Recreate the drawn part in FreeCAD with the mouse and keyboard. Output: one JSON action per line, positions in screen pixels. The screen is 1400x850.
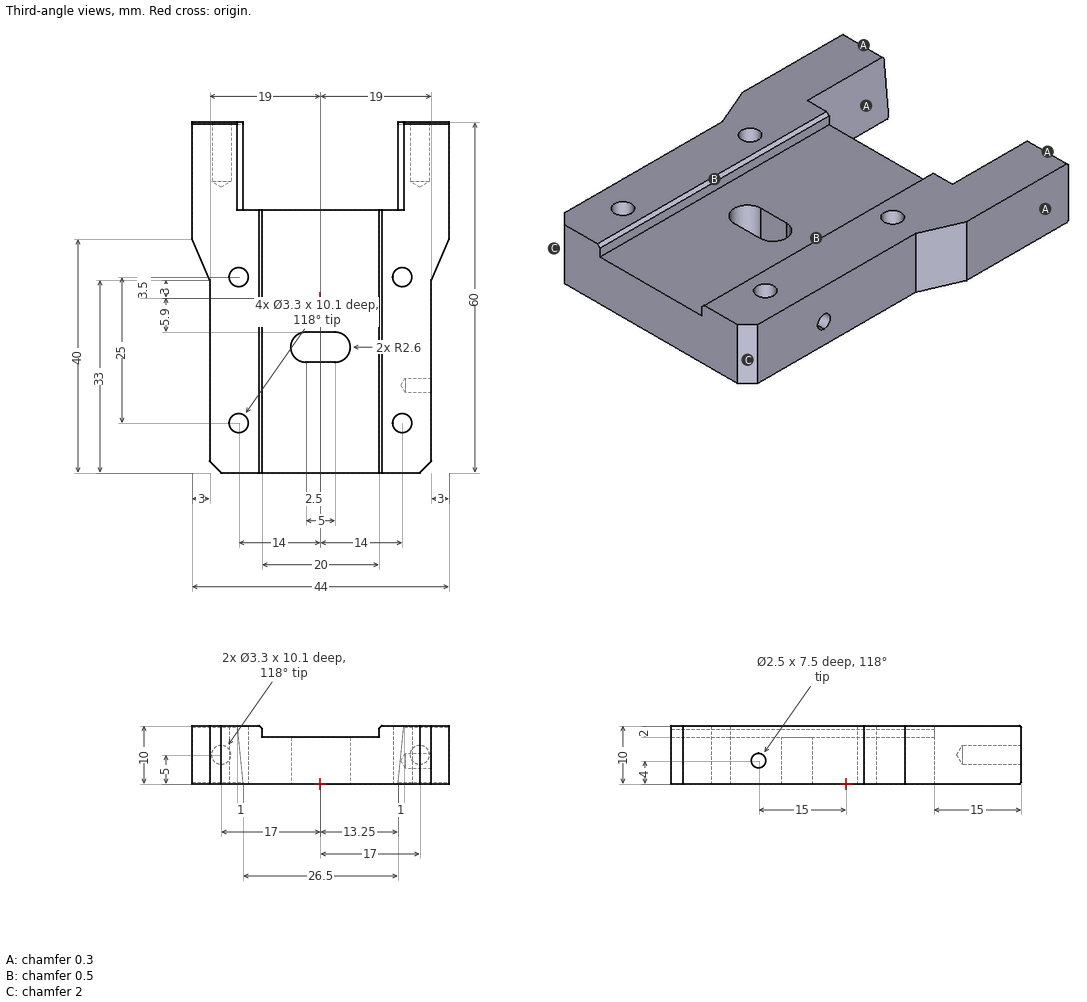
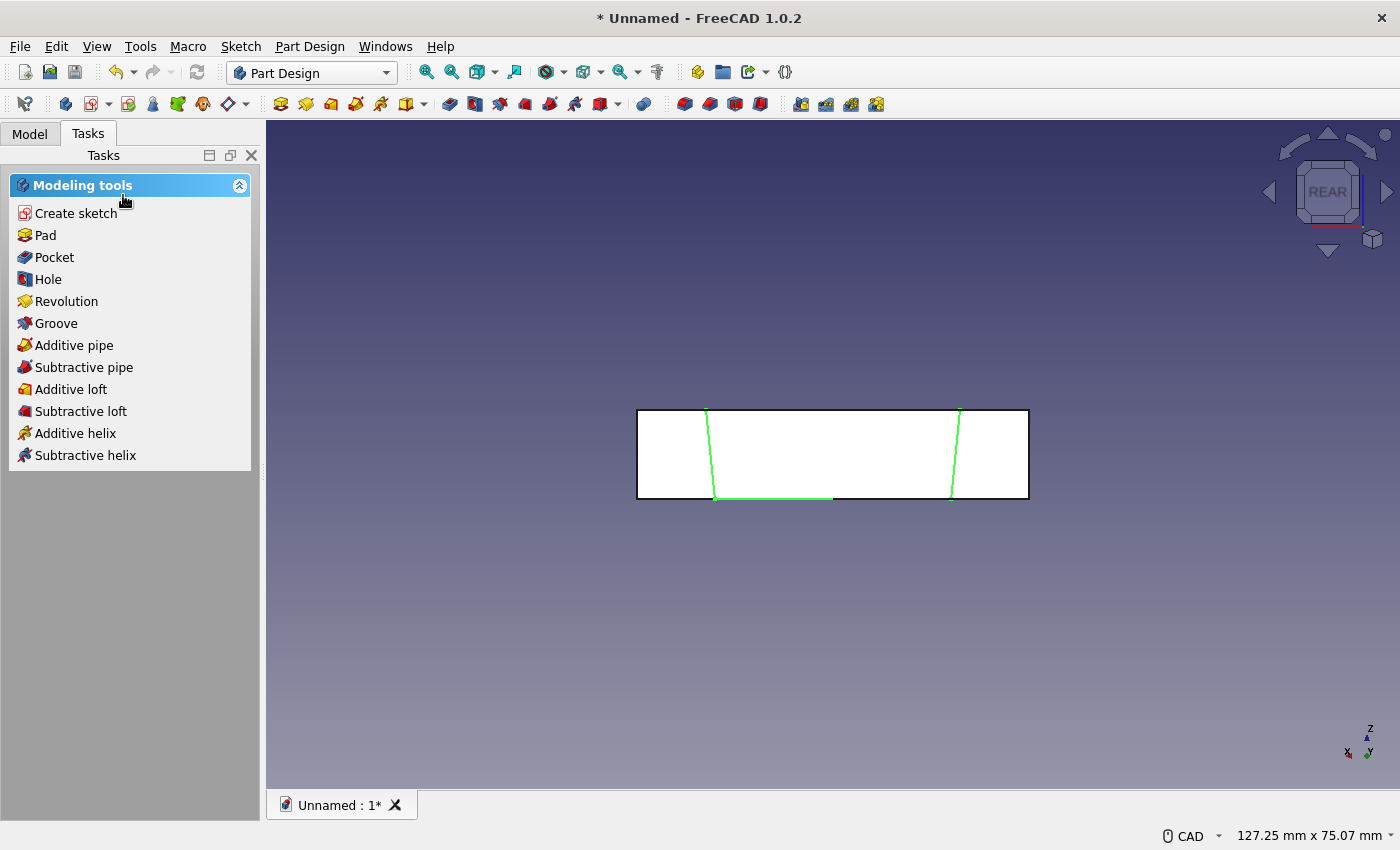
{"action": "left_click", "coordinate": [450, 104]}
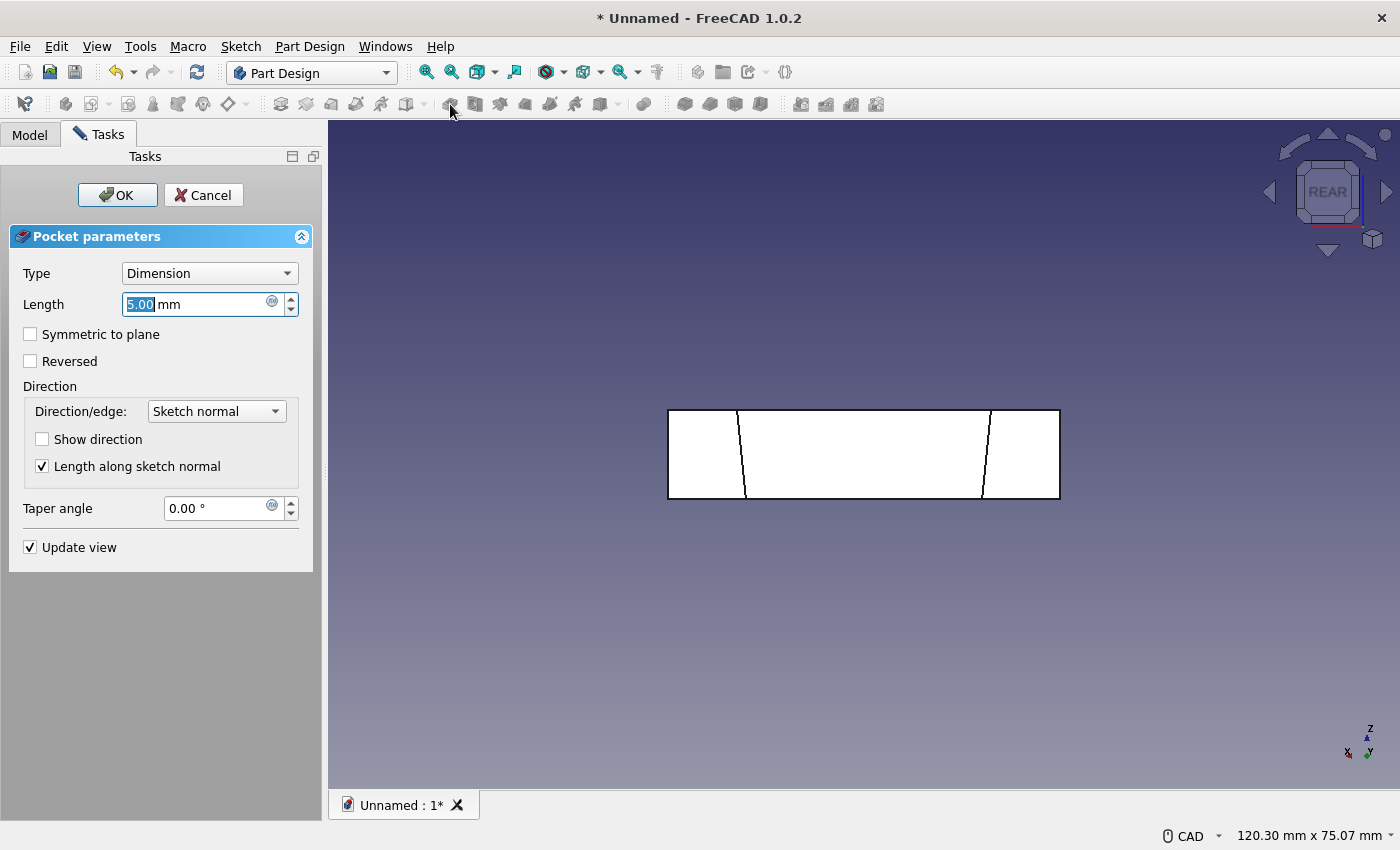
{"action": "type", "text": "15"}
{"action": "key", "text": "Tab"}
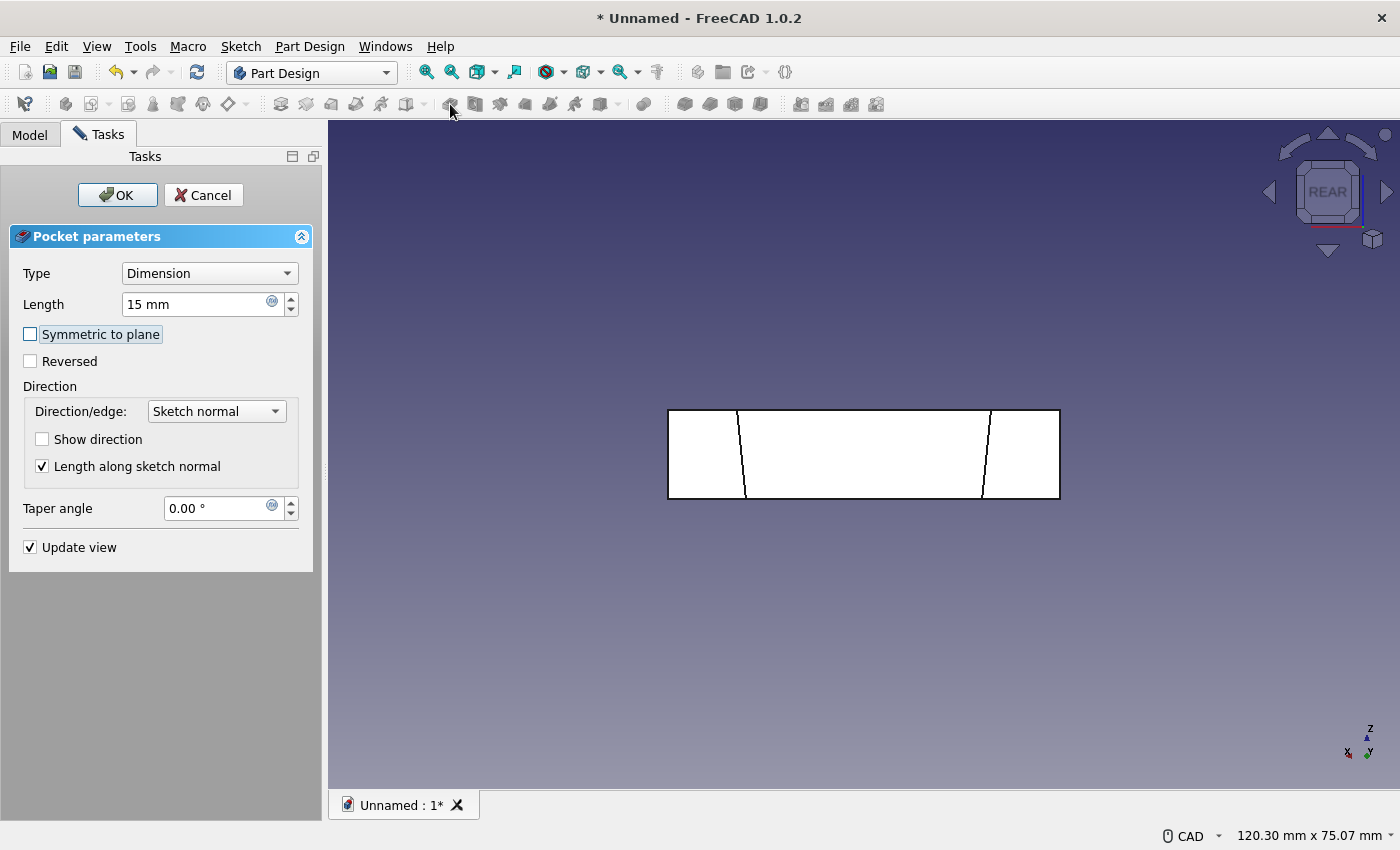
{"action": "left_click", "coordinate": [118, 195]}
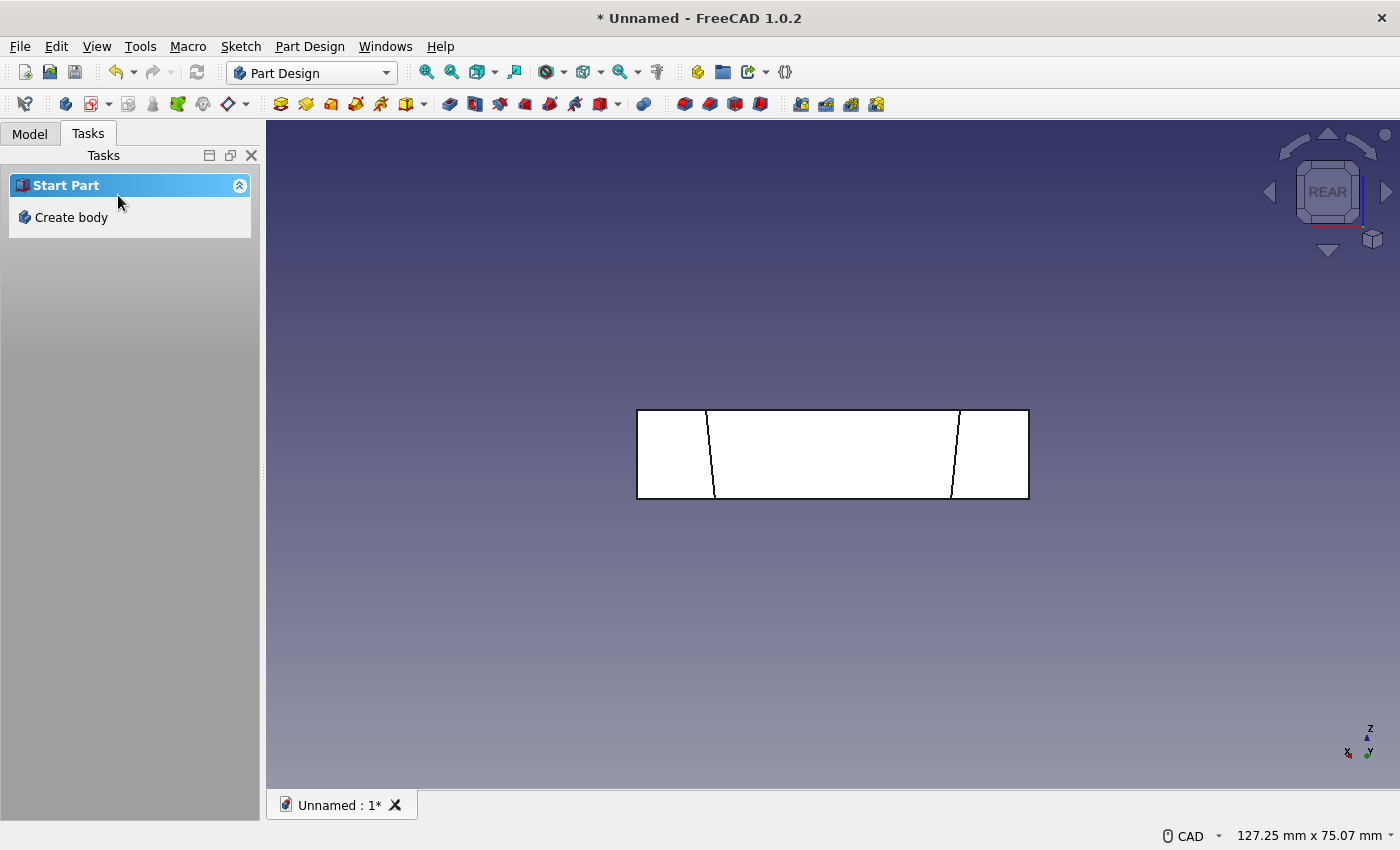
{"action": "left_click", "coordinate": [427, 72]}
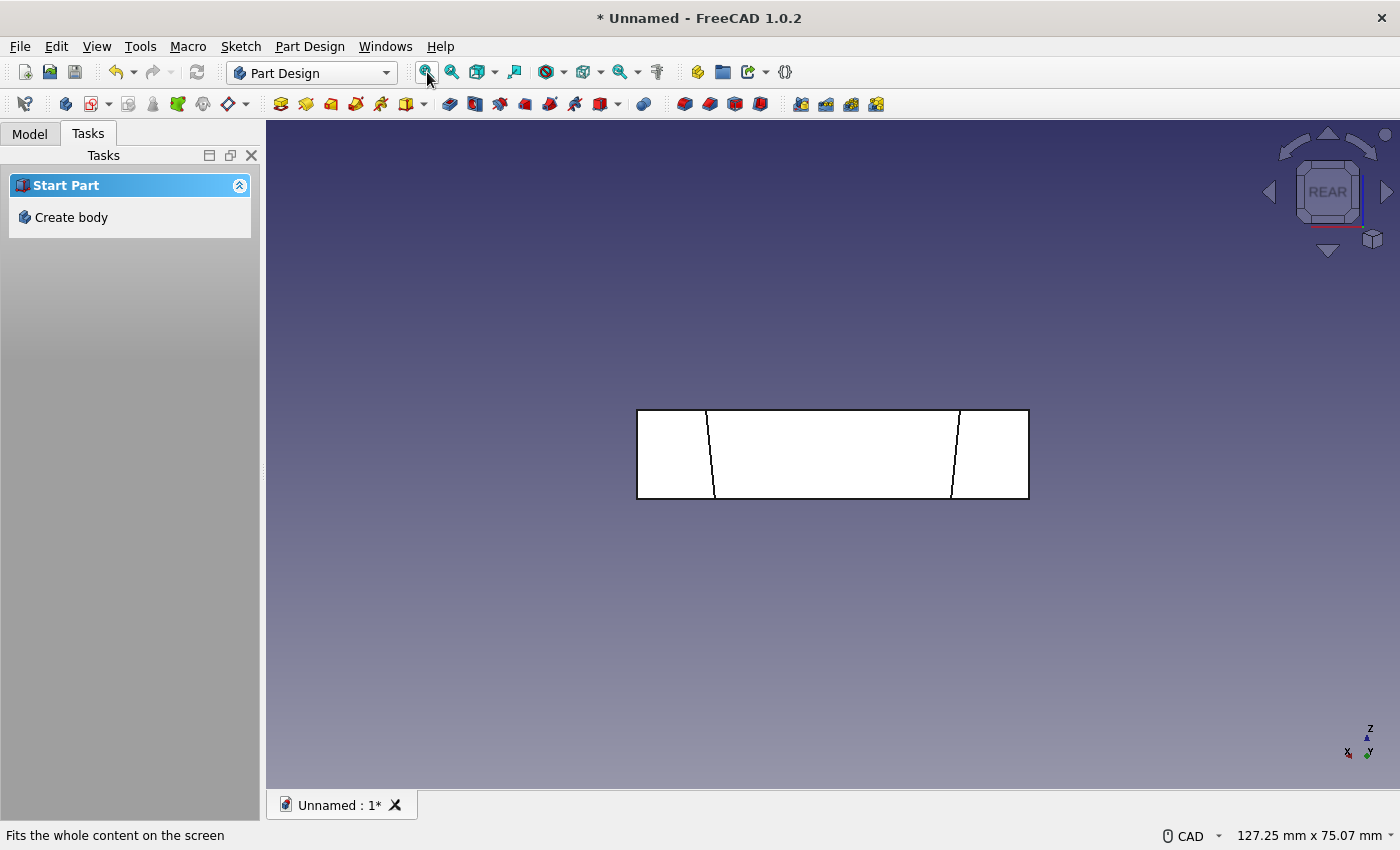
{"action": "key", "text": "0"}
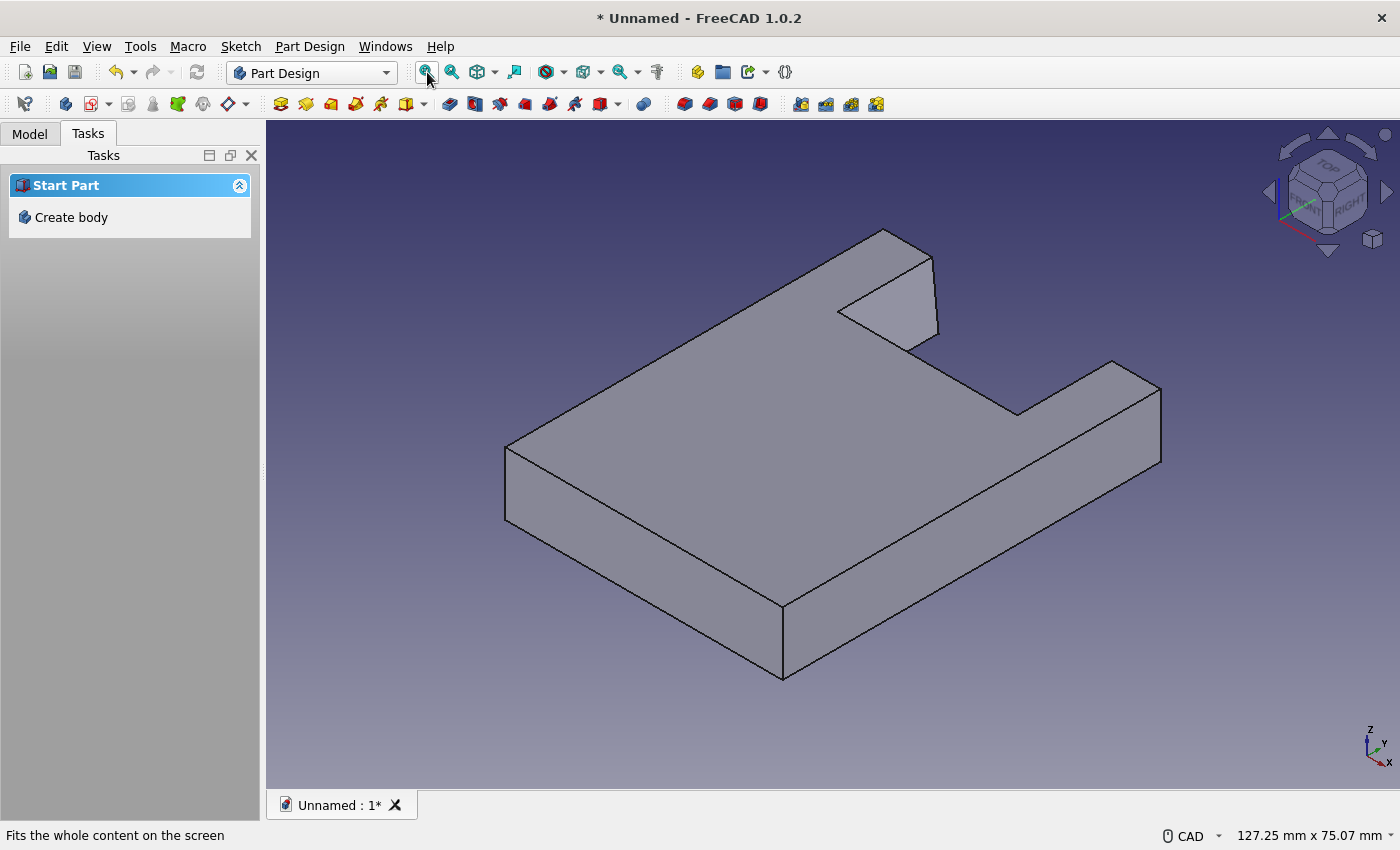
{"action": "left_click", "coordinate": [779, 448]}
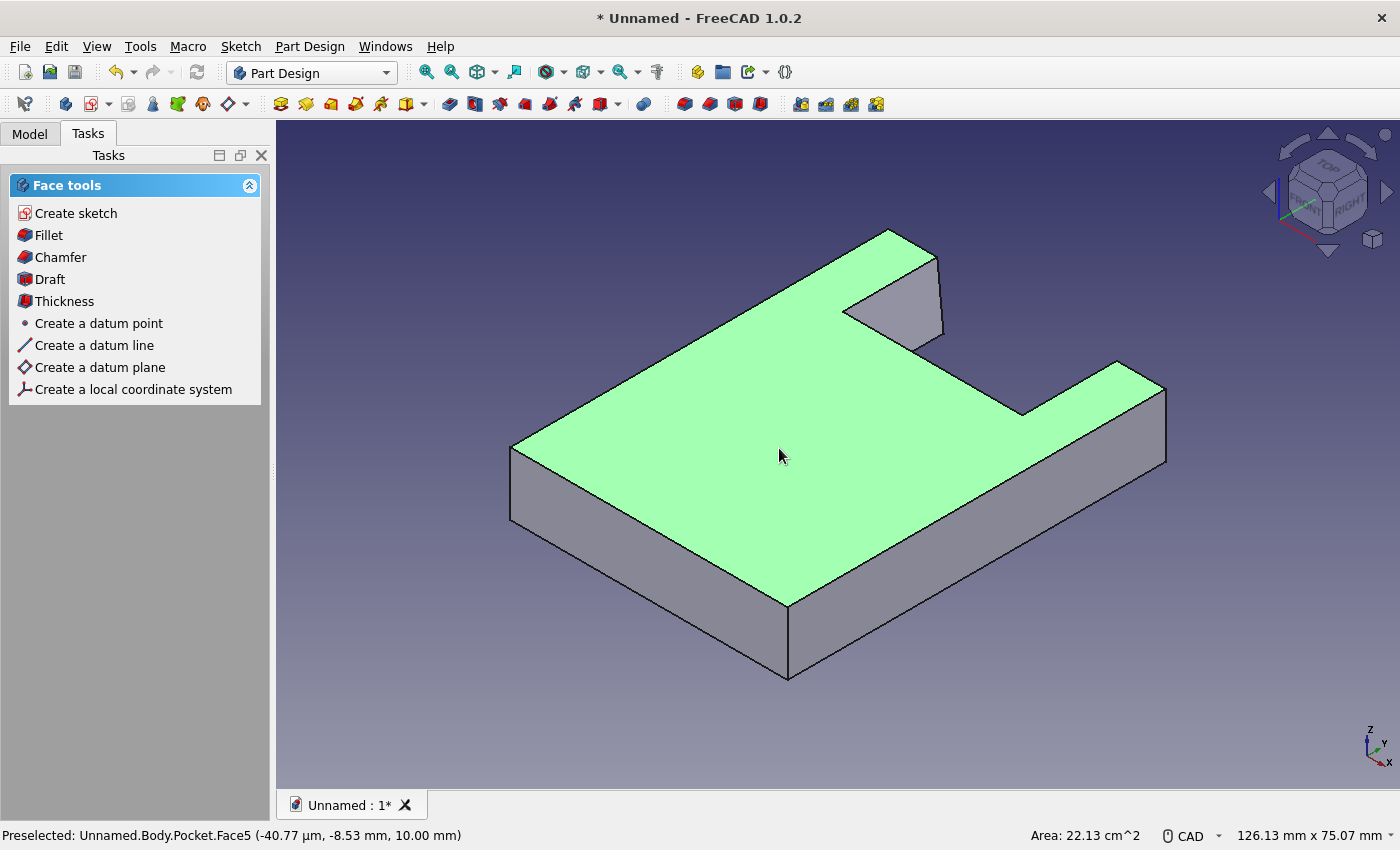
{"action": "left_click", "coordinate": [90, 104]}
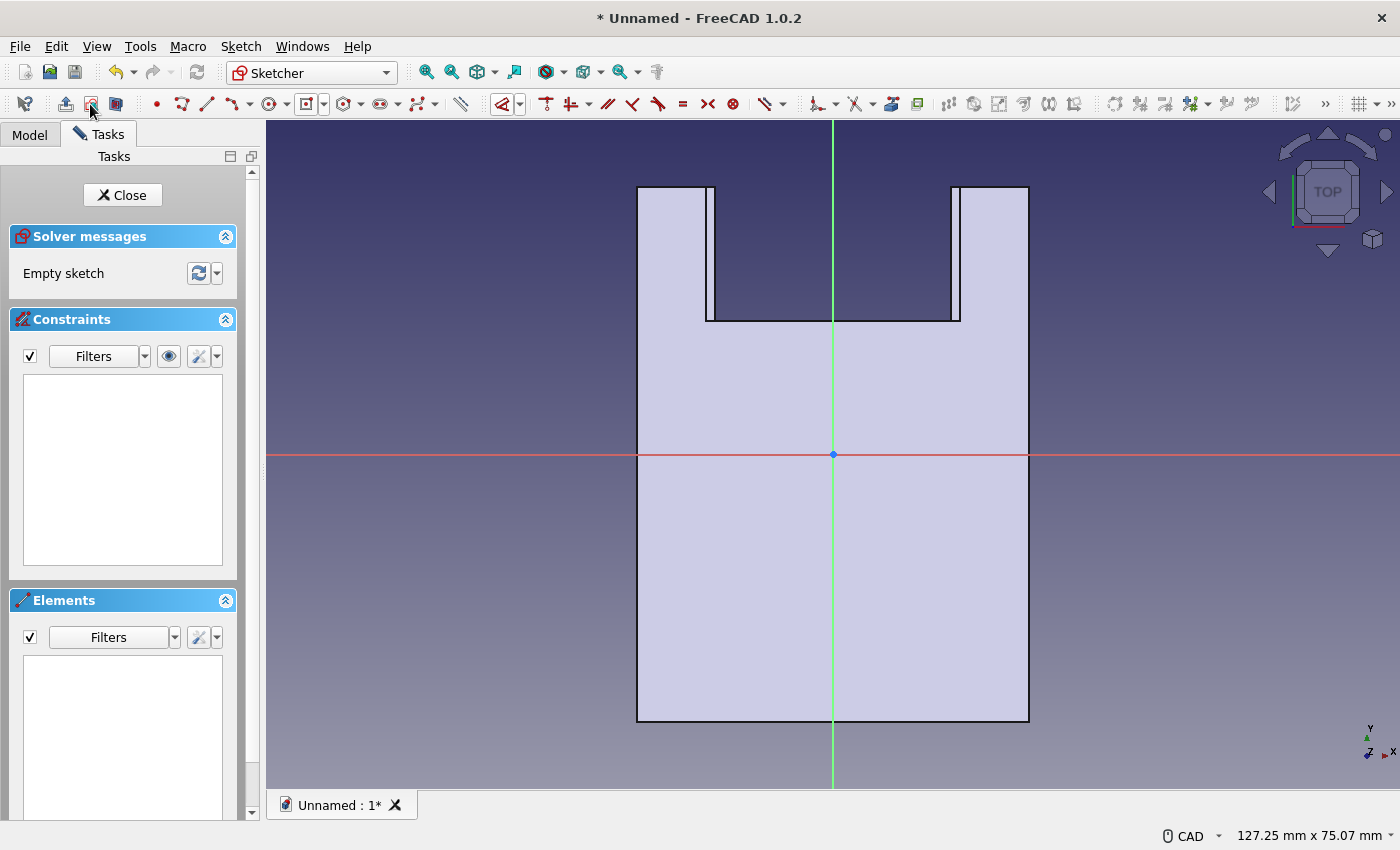
{"action": "key", "text": "g v"}